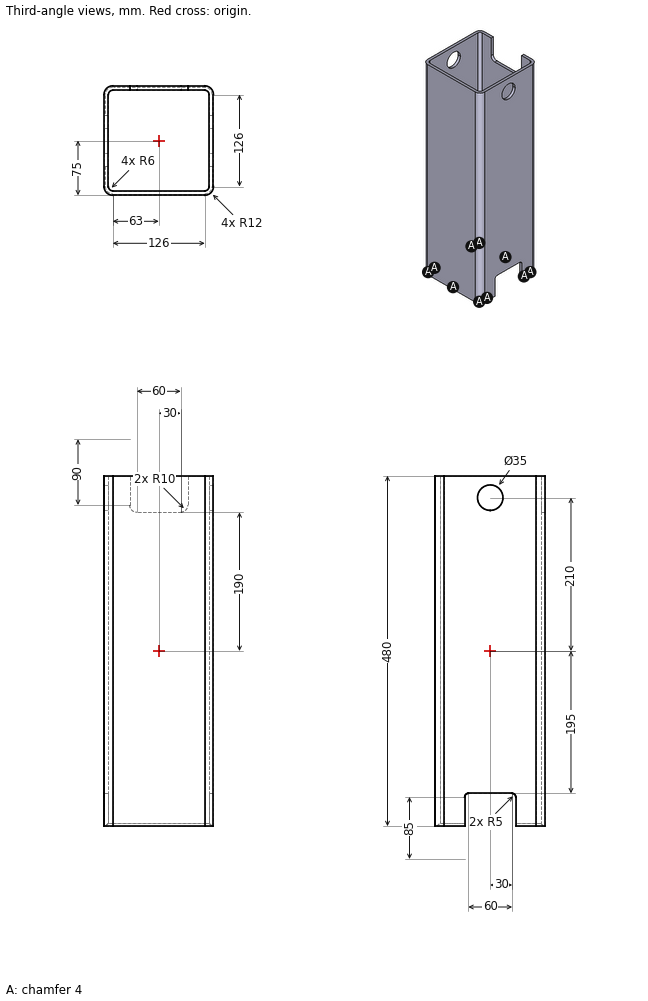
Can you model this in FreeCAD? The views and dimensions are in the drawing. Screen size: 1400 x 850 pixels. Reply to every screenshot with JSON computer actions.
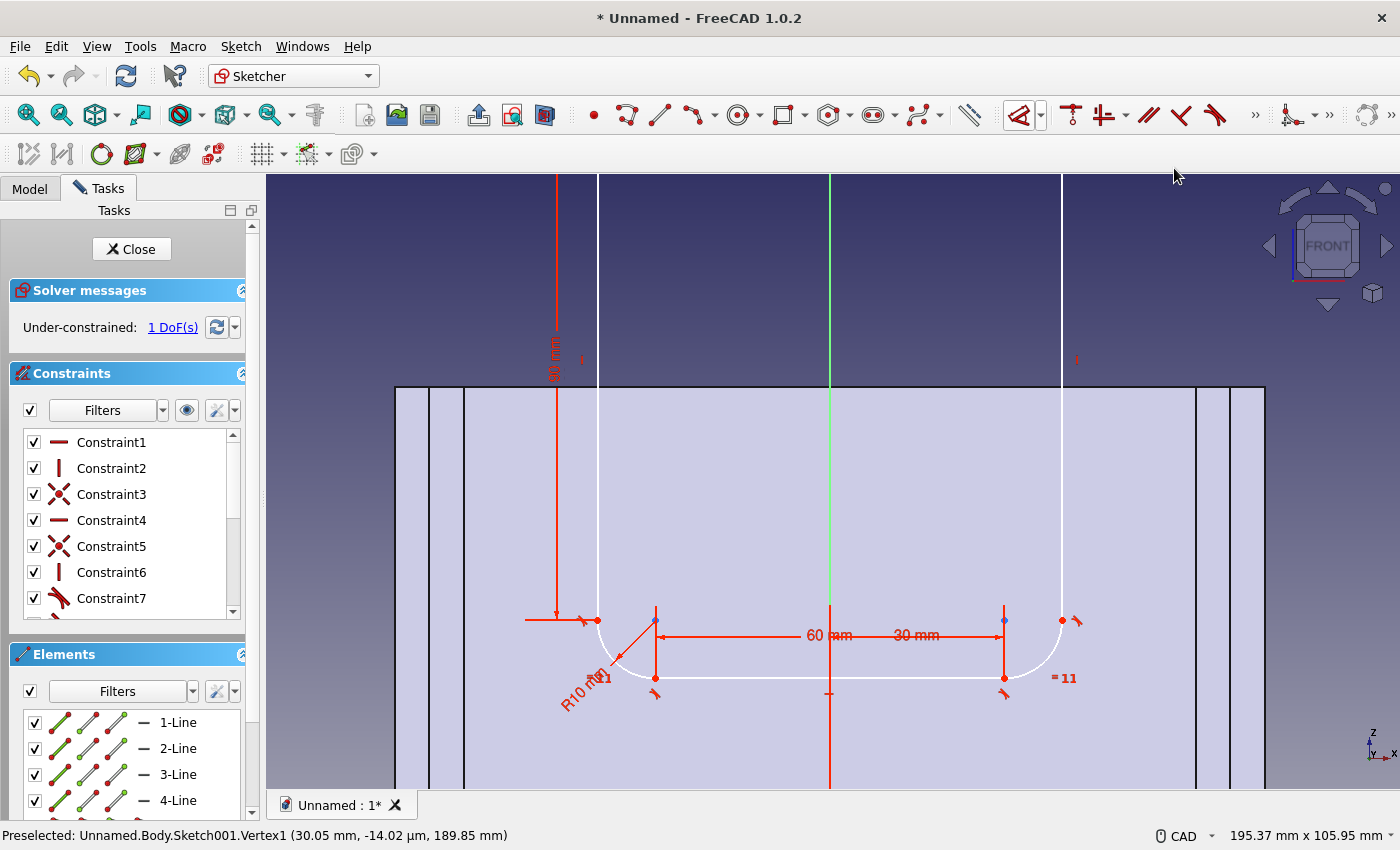
{"action": "left_click", "coordinate": [1004, 678]}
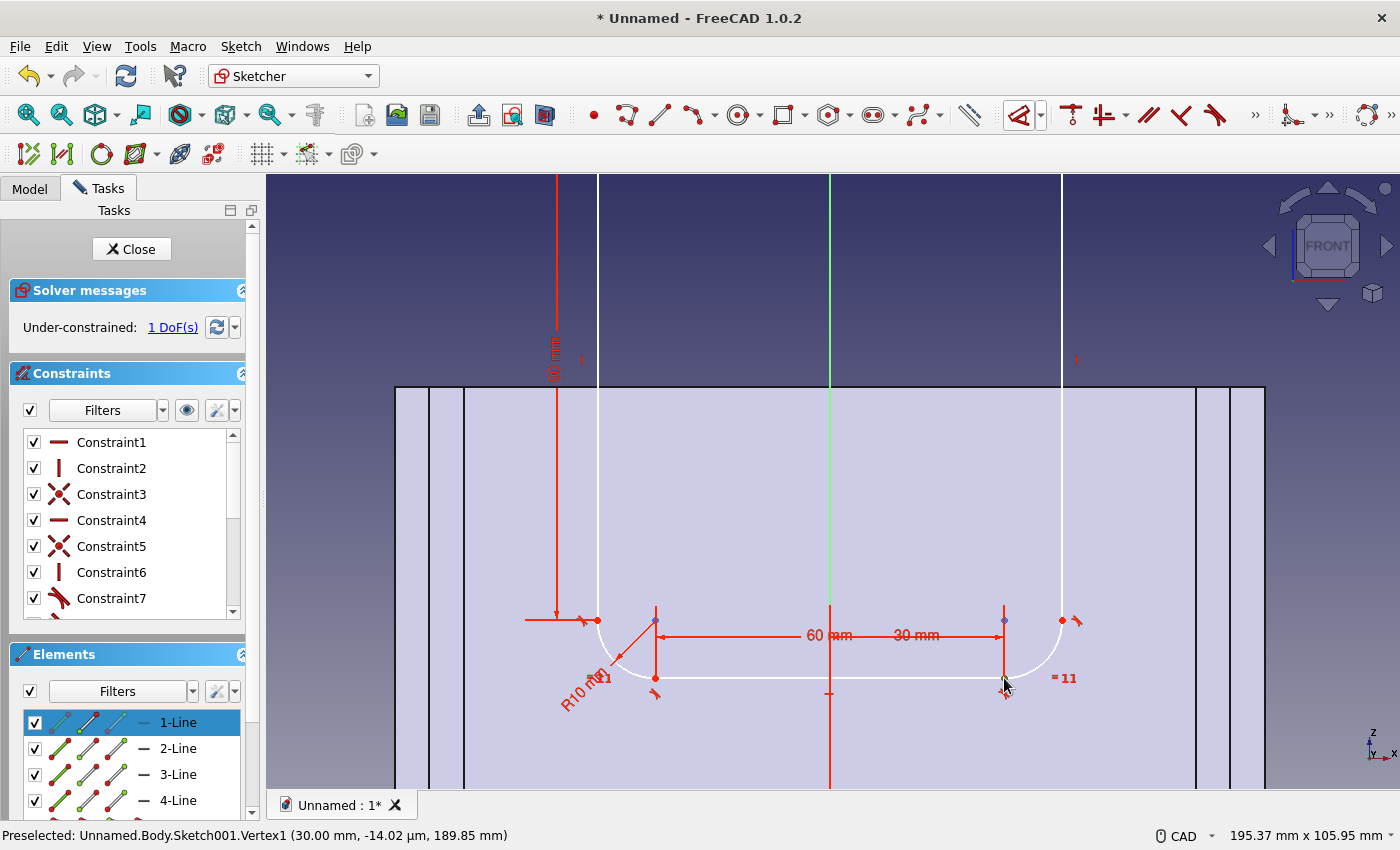
{"action": "key", "text": "i"}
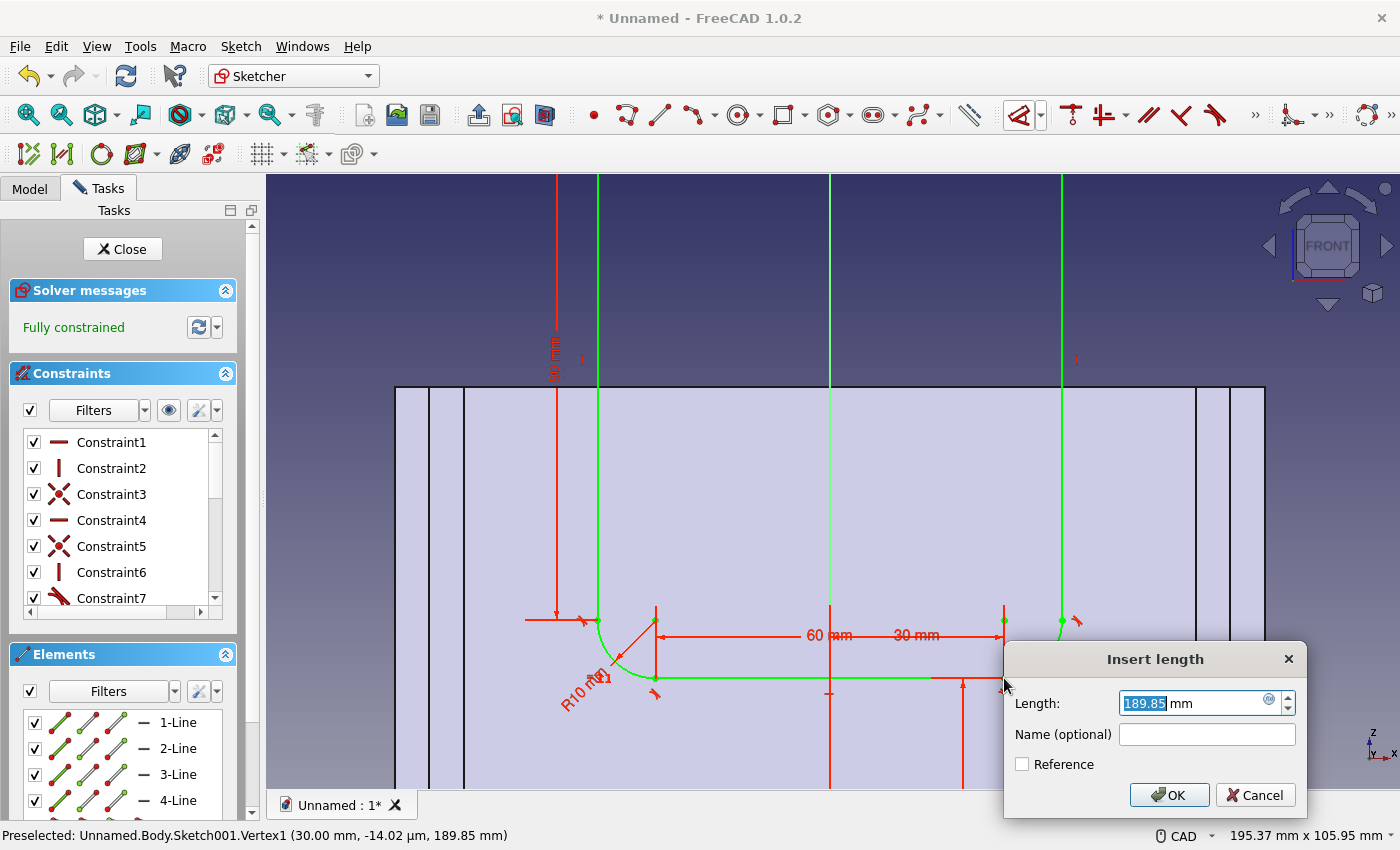
{"action": "type", "text": "190"}
{"action": "key", "text": "Return"}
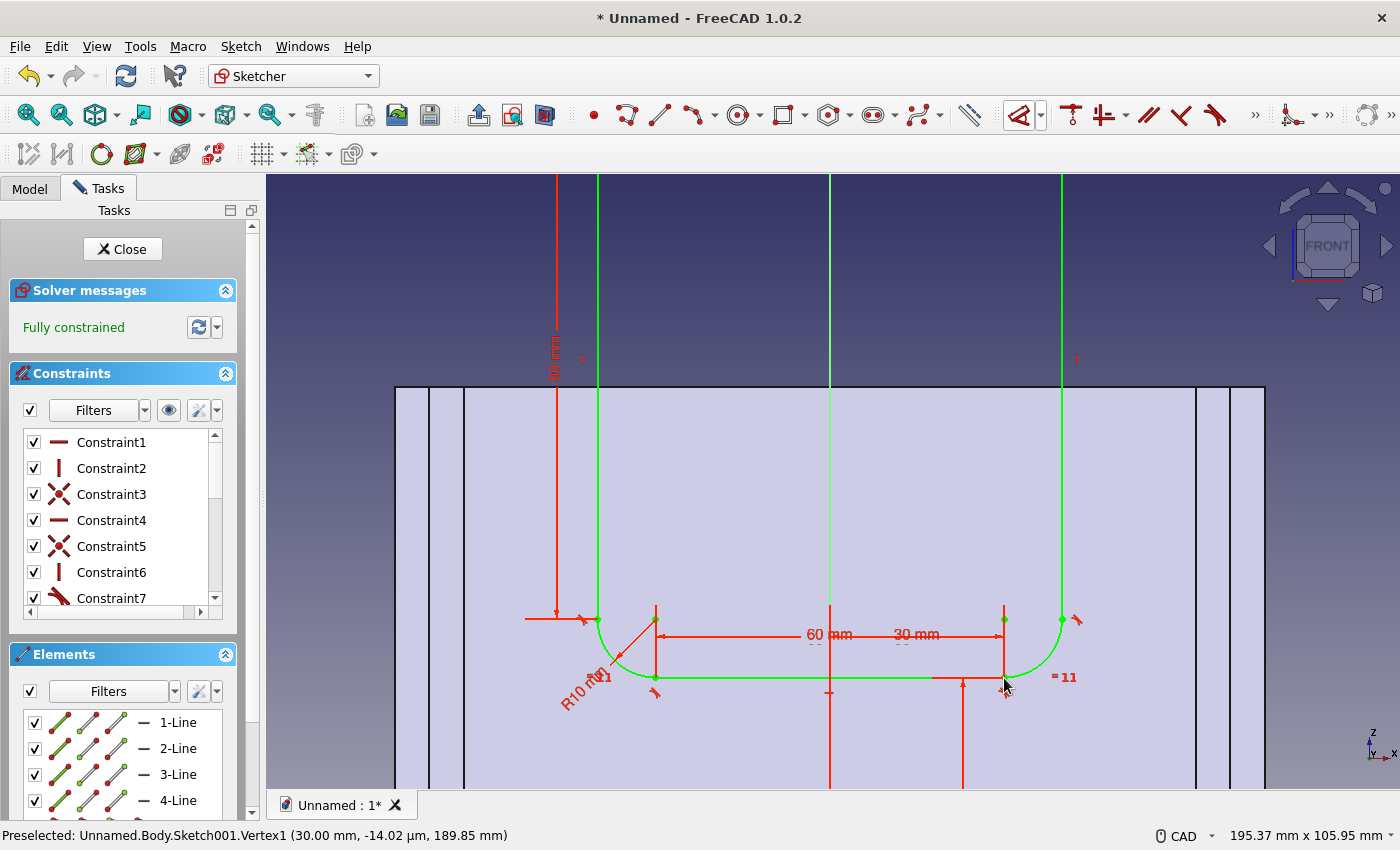
{"action": "left_click", "coordinate": [123, 249]}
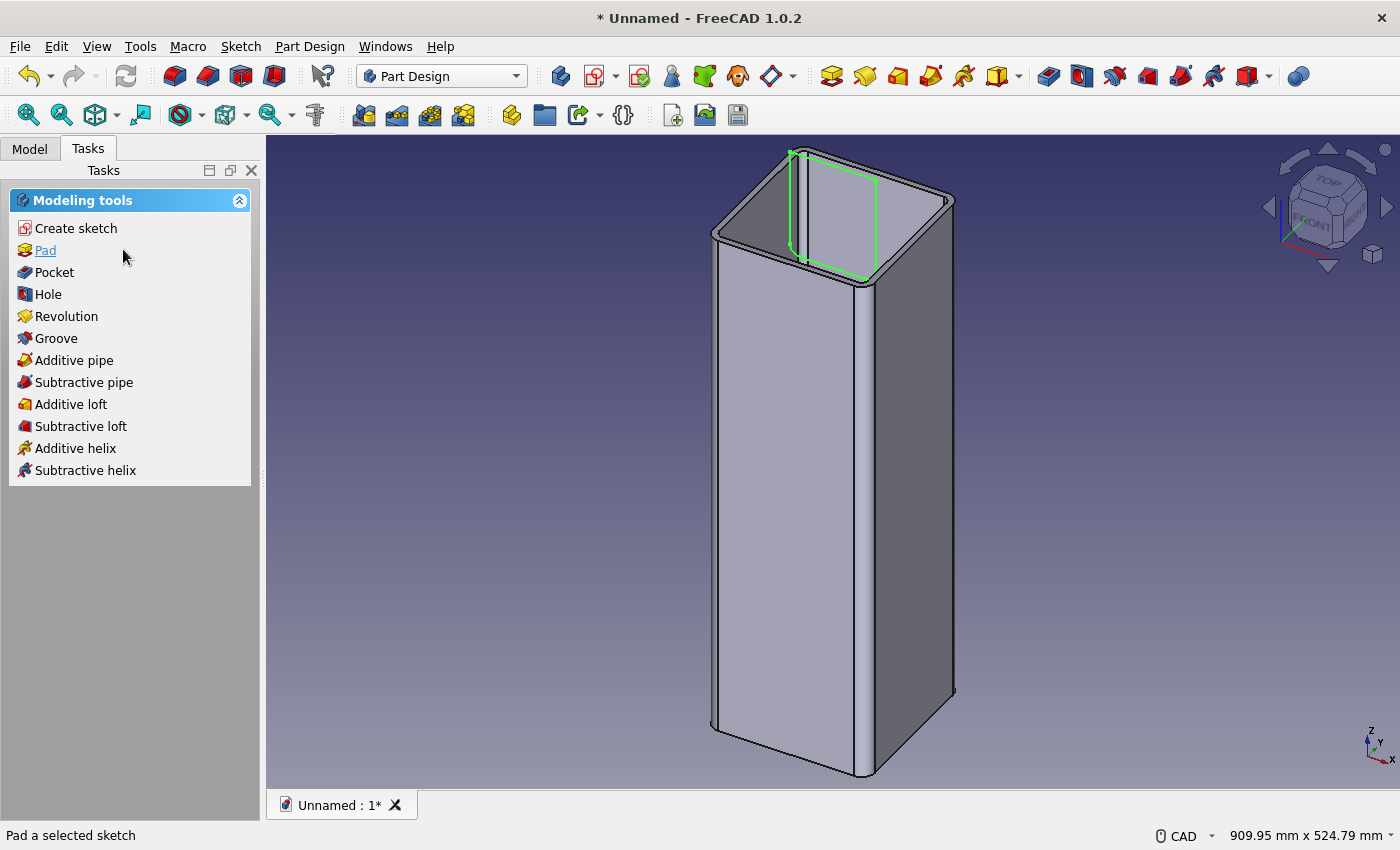
{"action": "left_click", "coordinate": [1049, 76]}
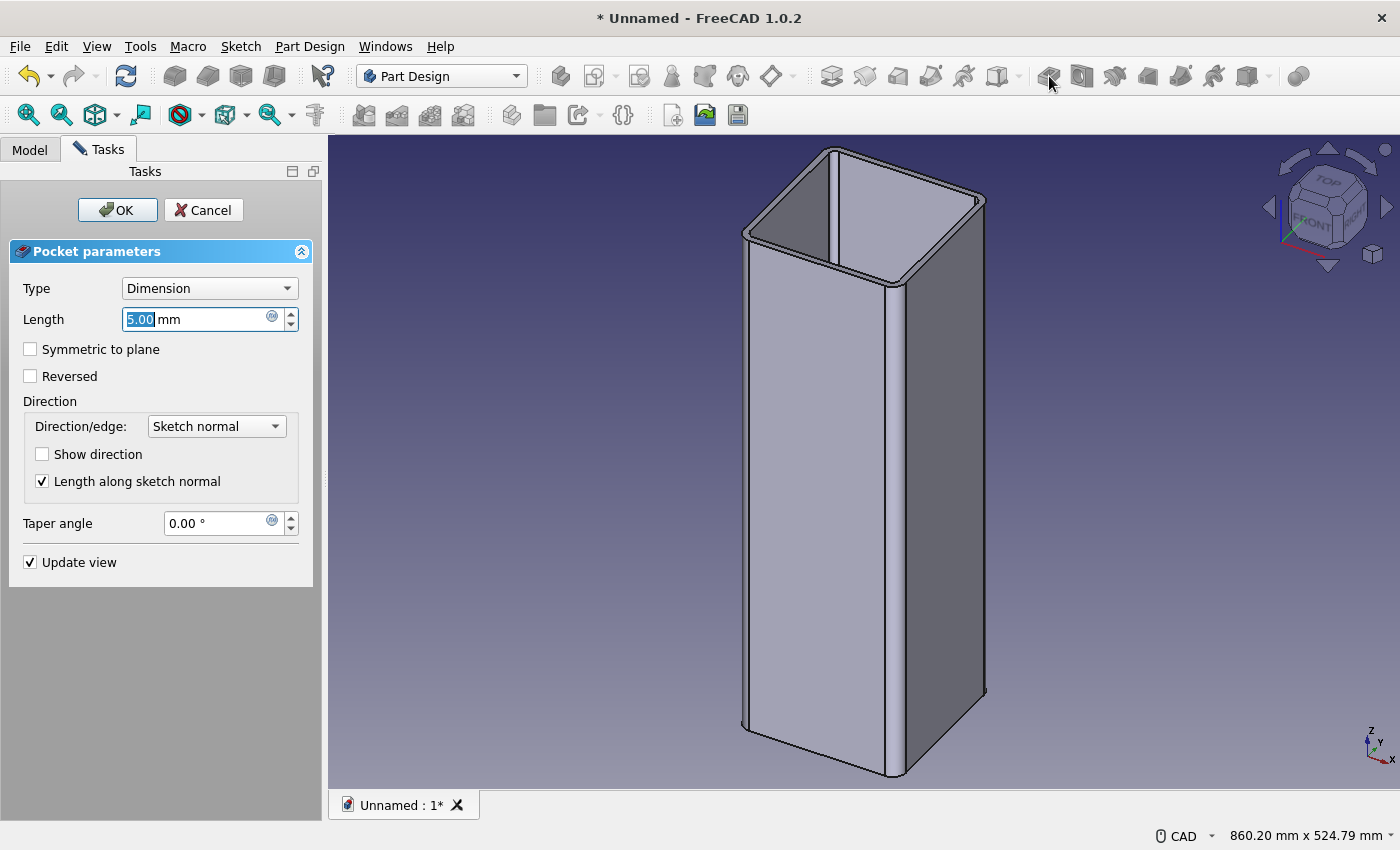
{"action": "left_click", "coordinate": [210, 288]}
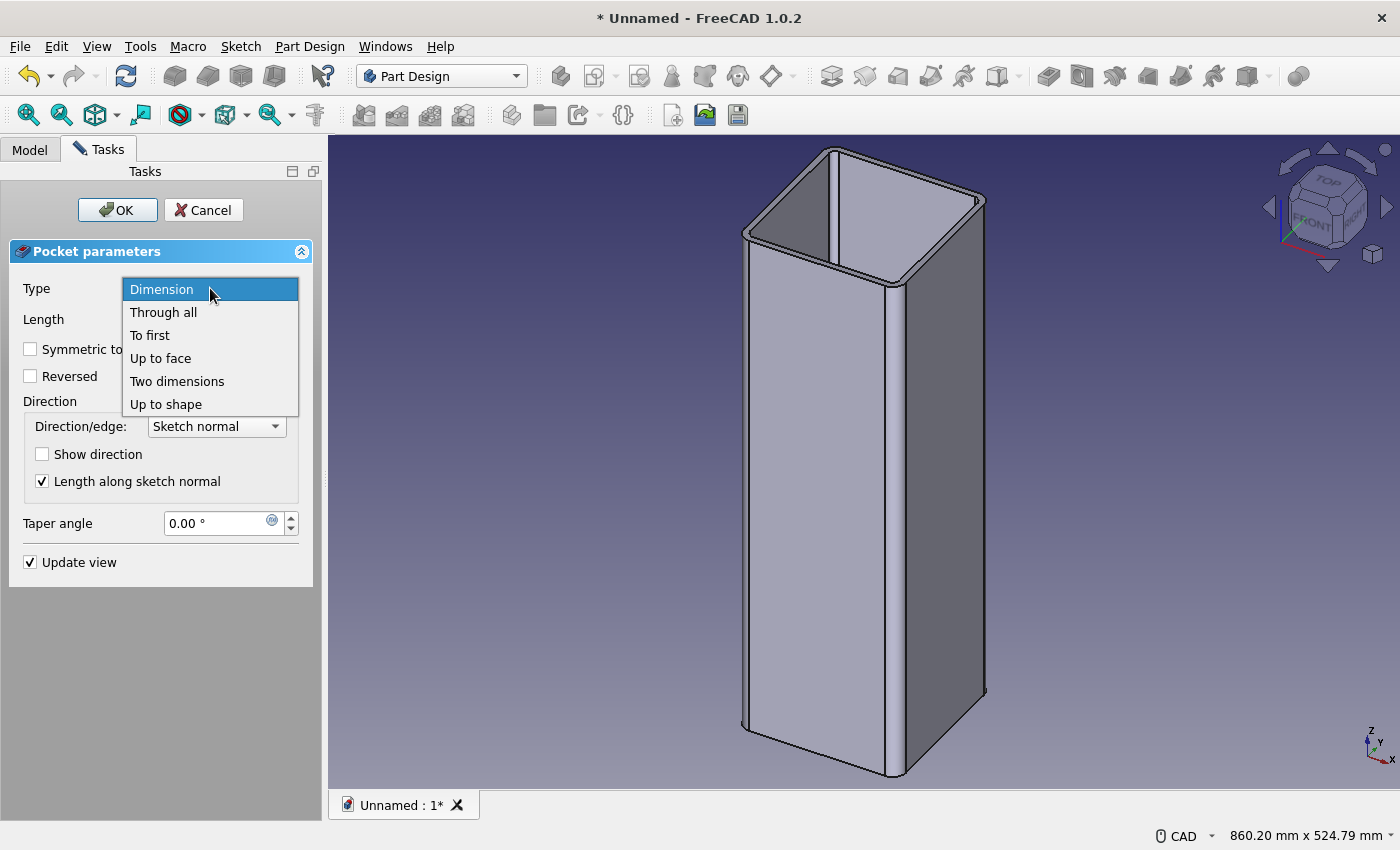
{"action": "left_click", "coordinate": [208, 312]}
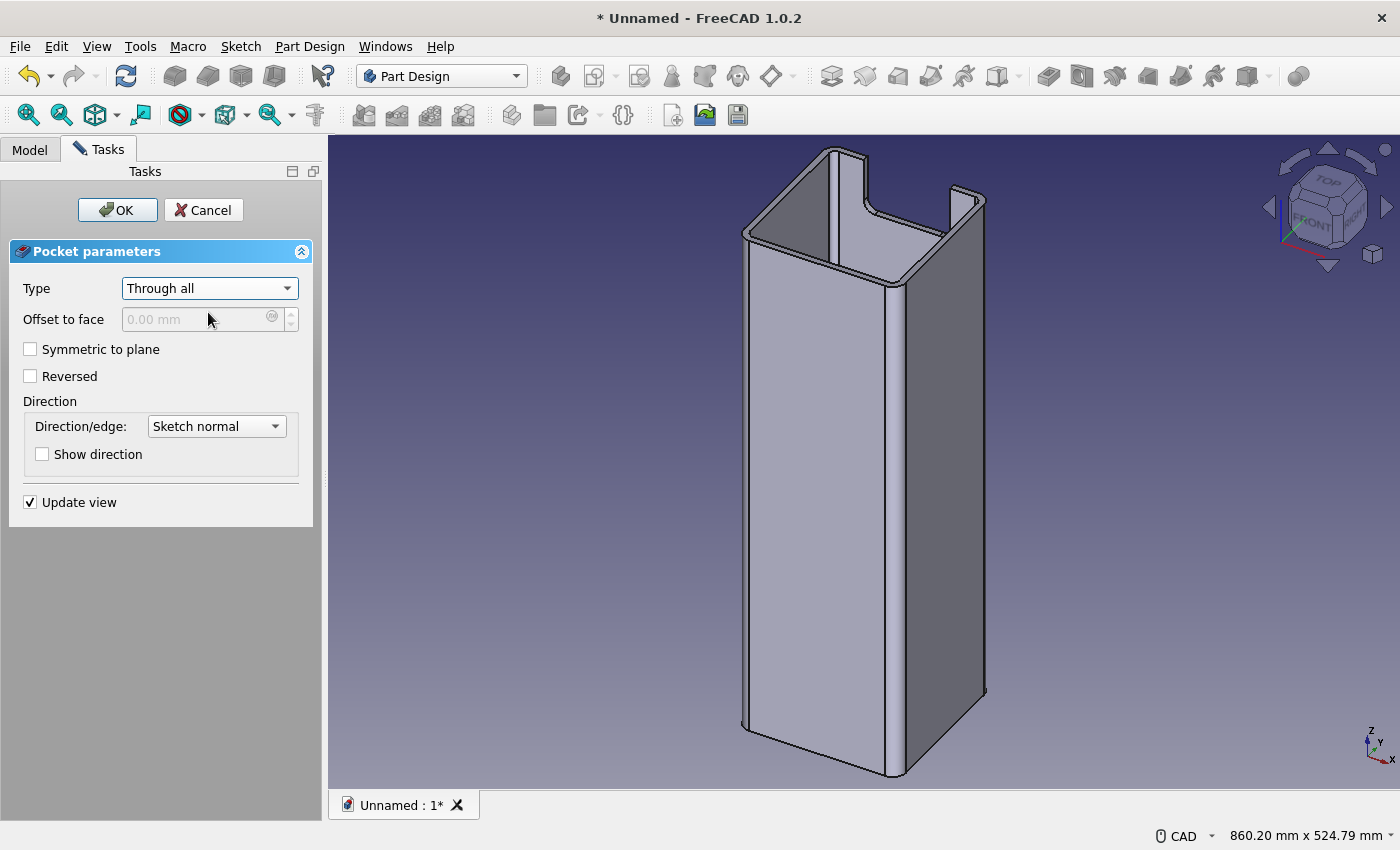
{"action": "left_click", "coordinate": [118, 210]}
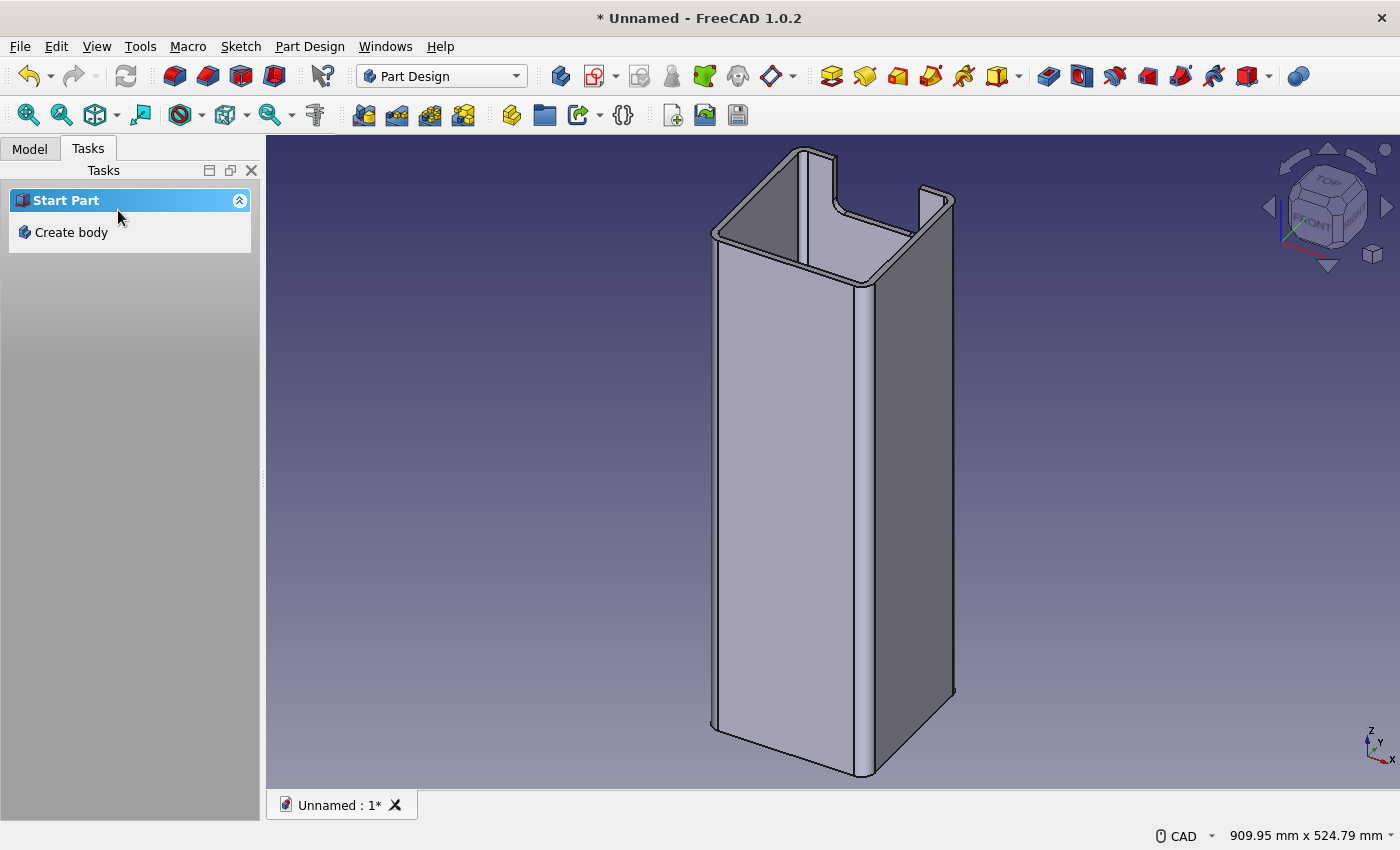
{"action": "left_click", "coordinate": [594, 76]}